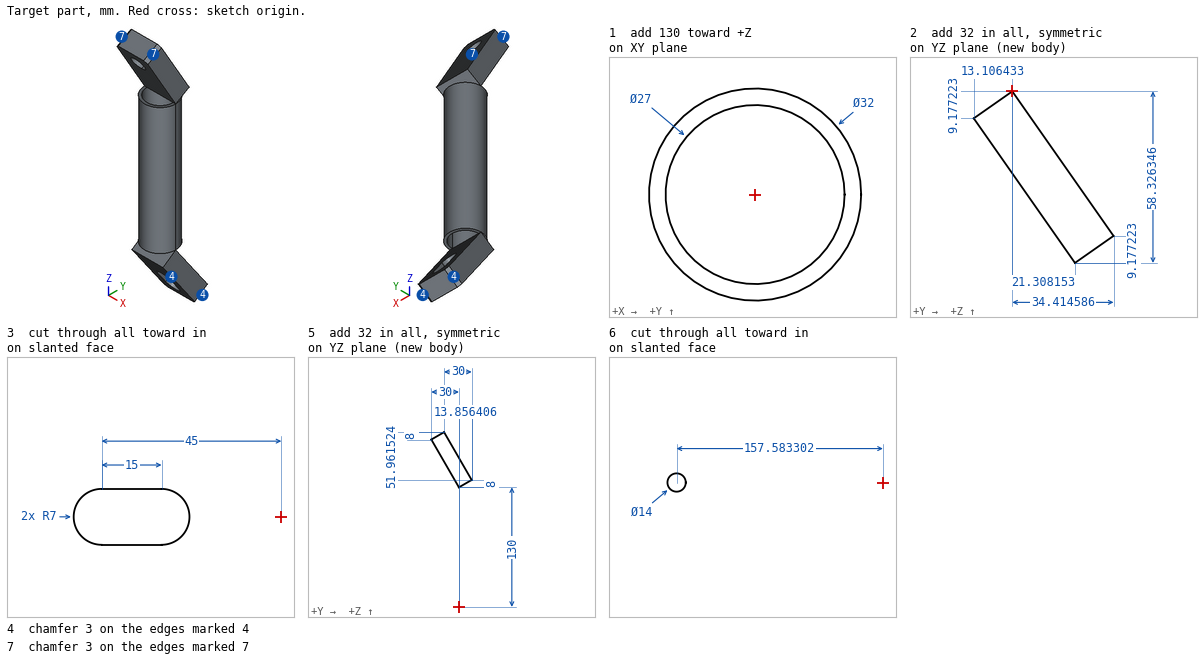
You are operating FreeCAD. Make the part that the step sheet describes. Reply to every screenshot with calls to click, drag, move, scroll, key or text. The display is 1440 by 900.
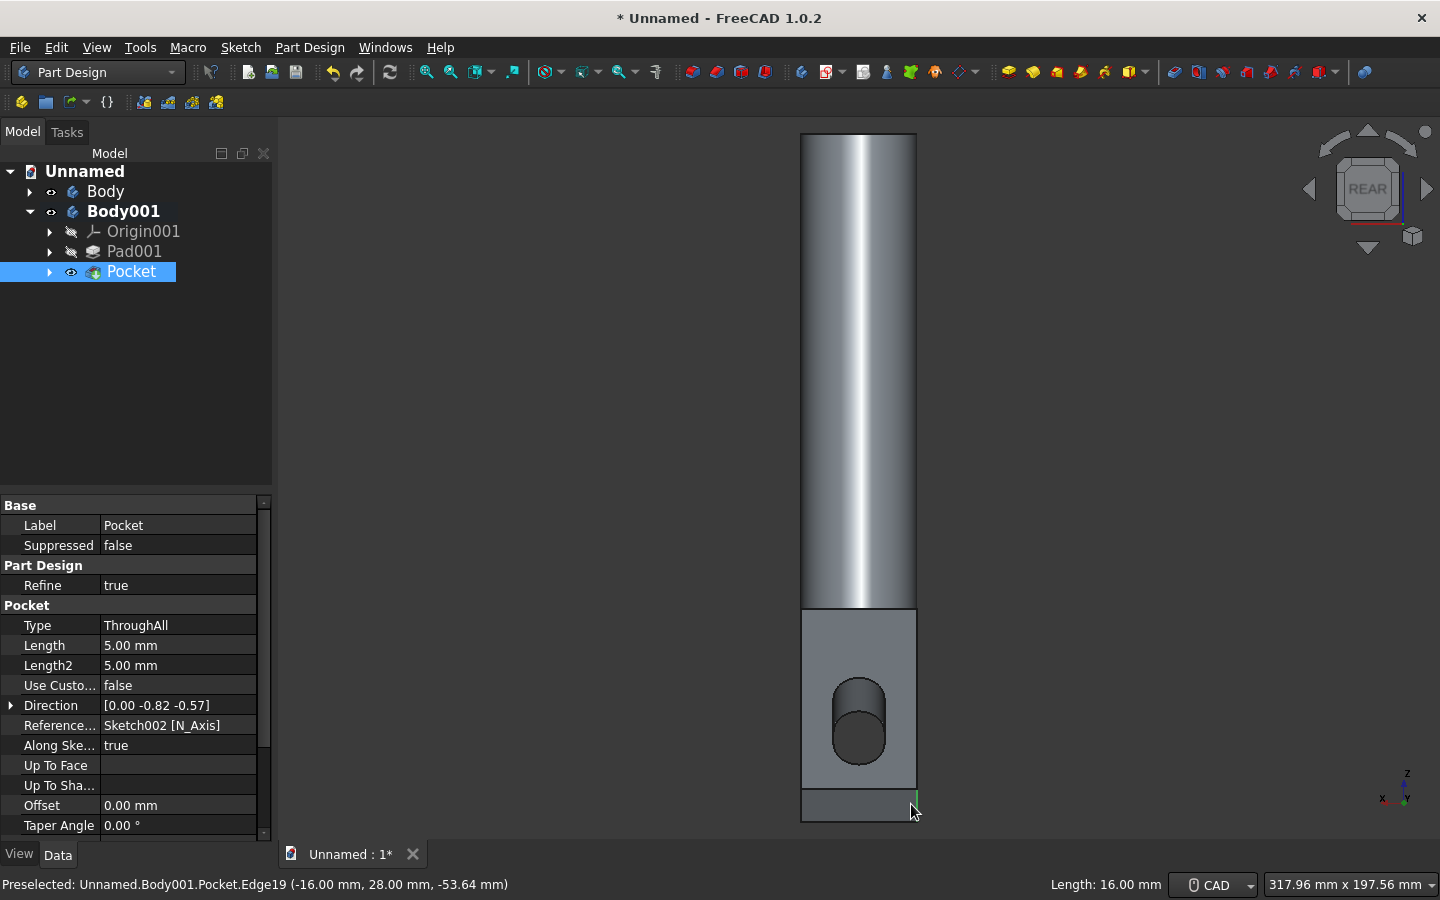
key(0)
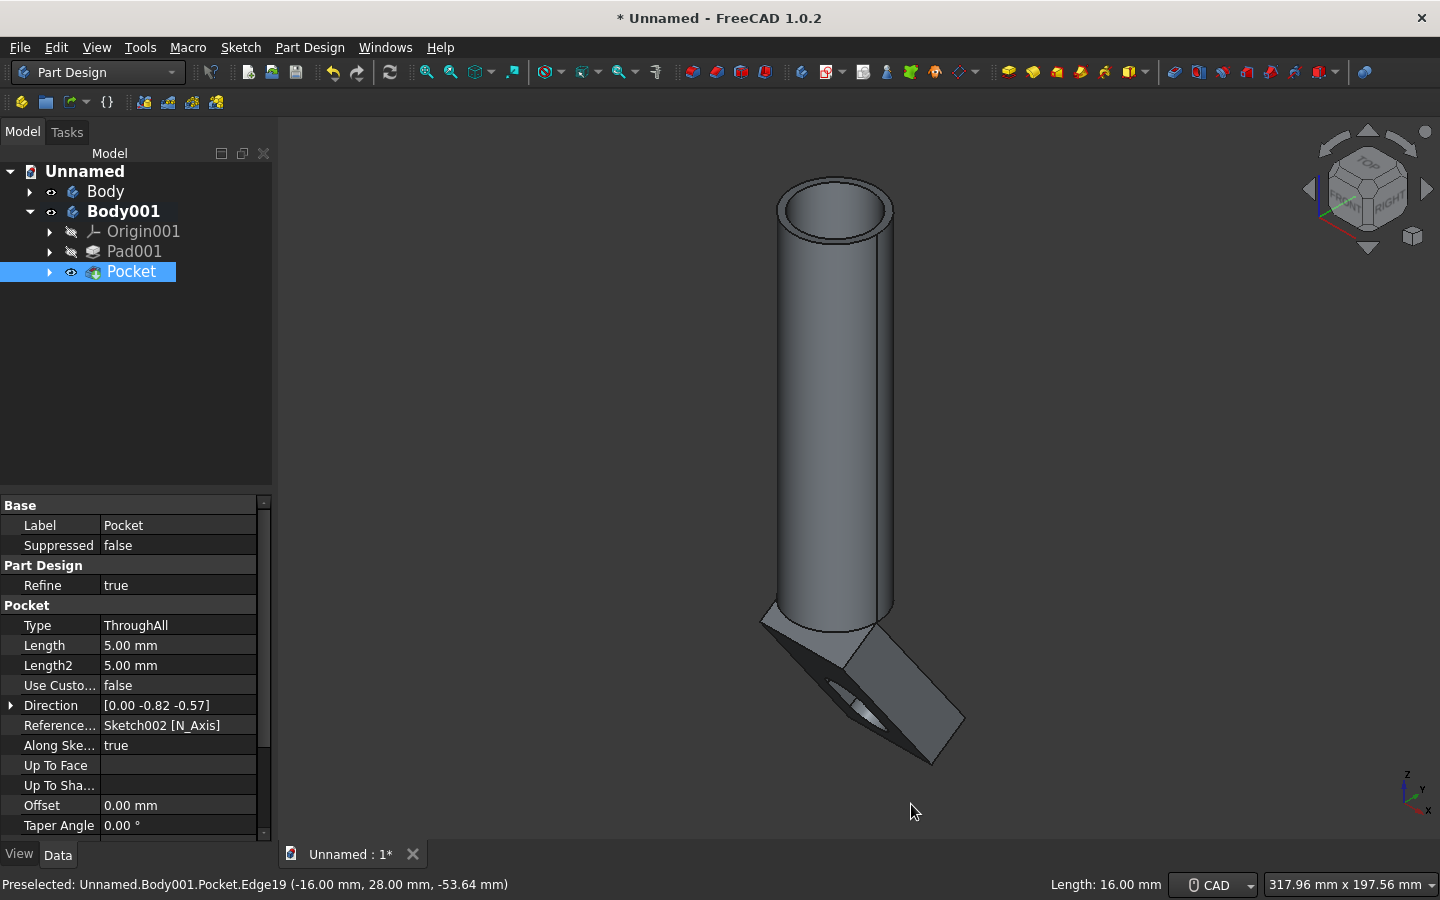
key(v)
key(f)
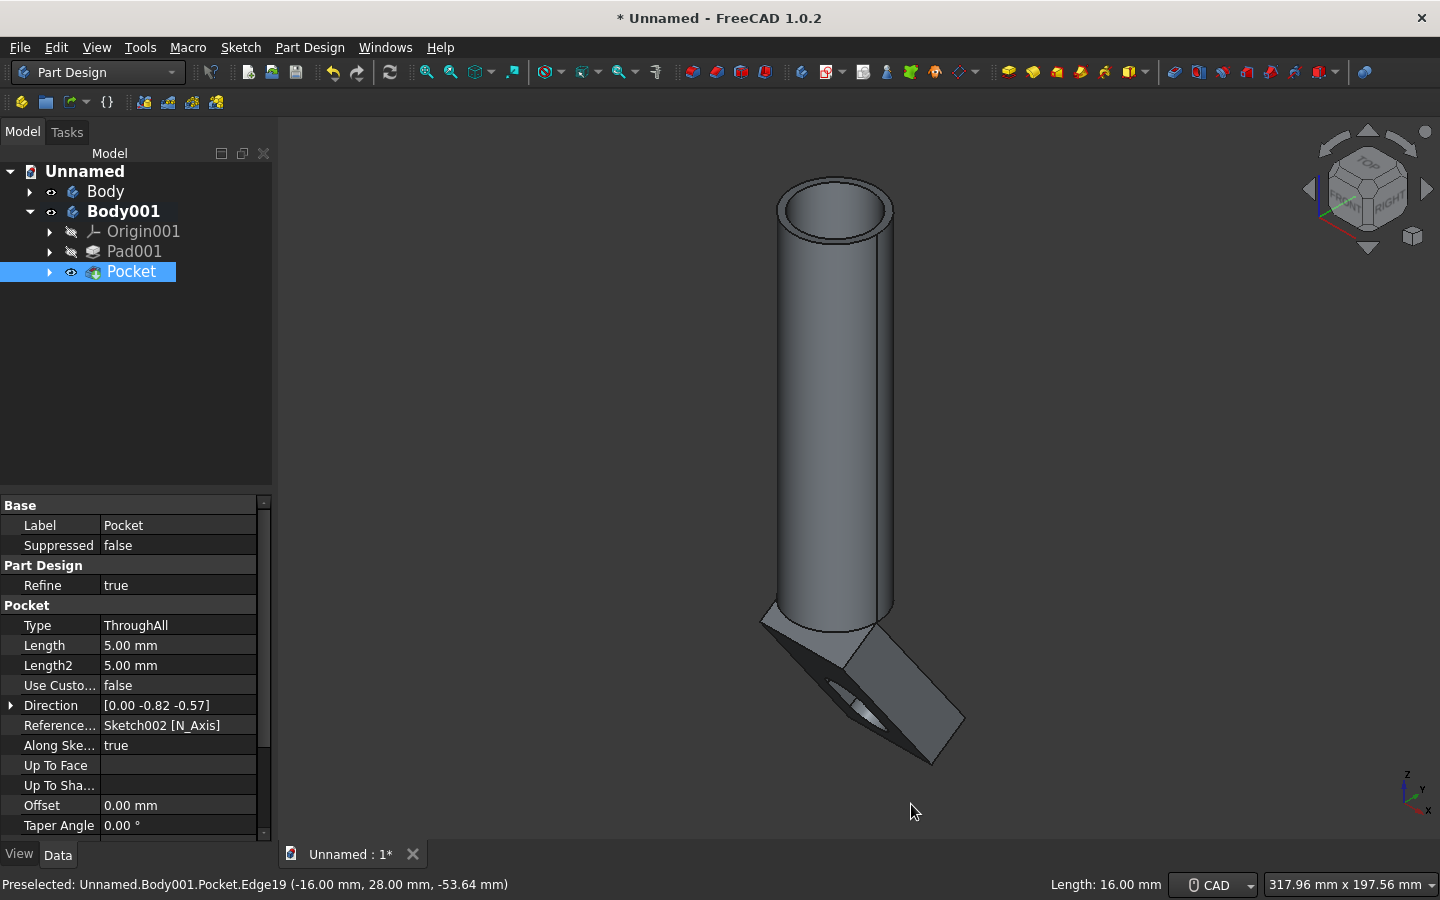
key(2)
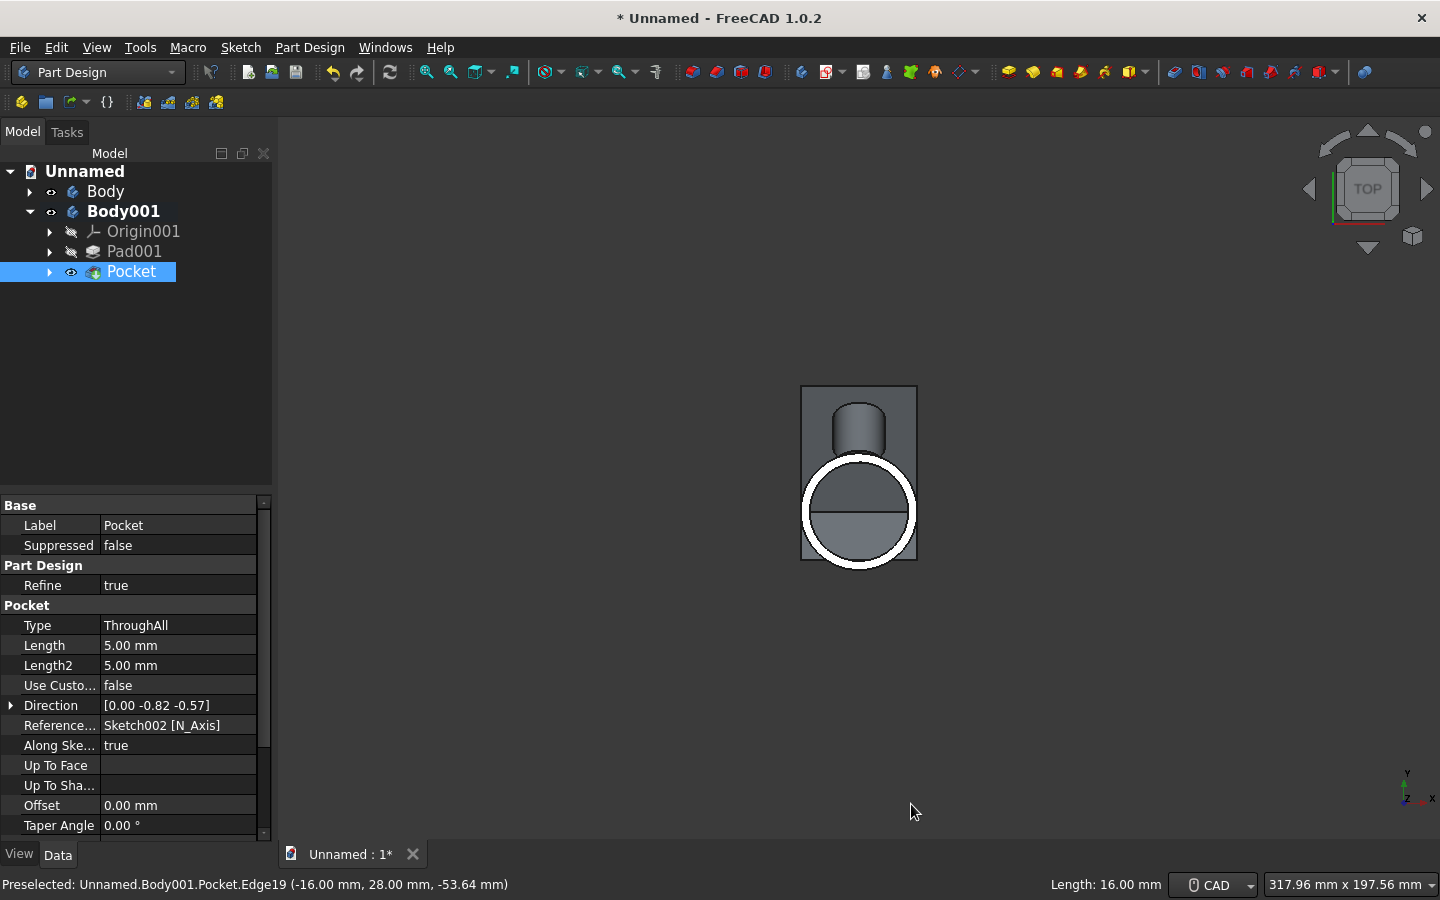
click(428, 72)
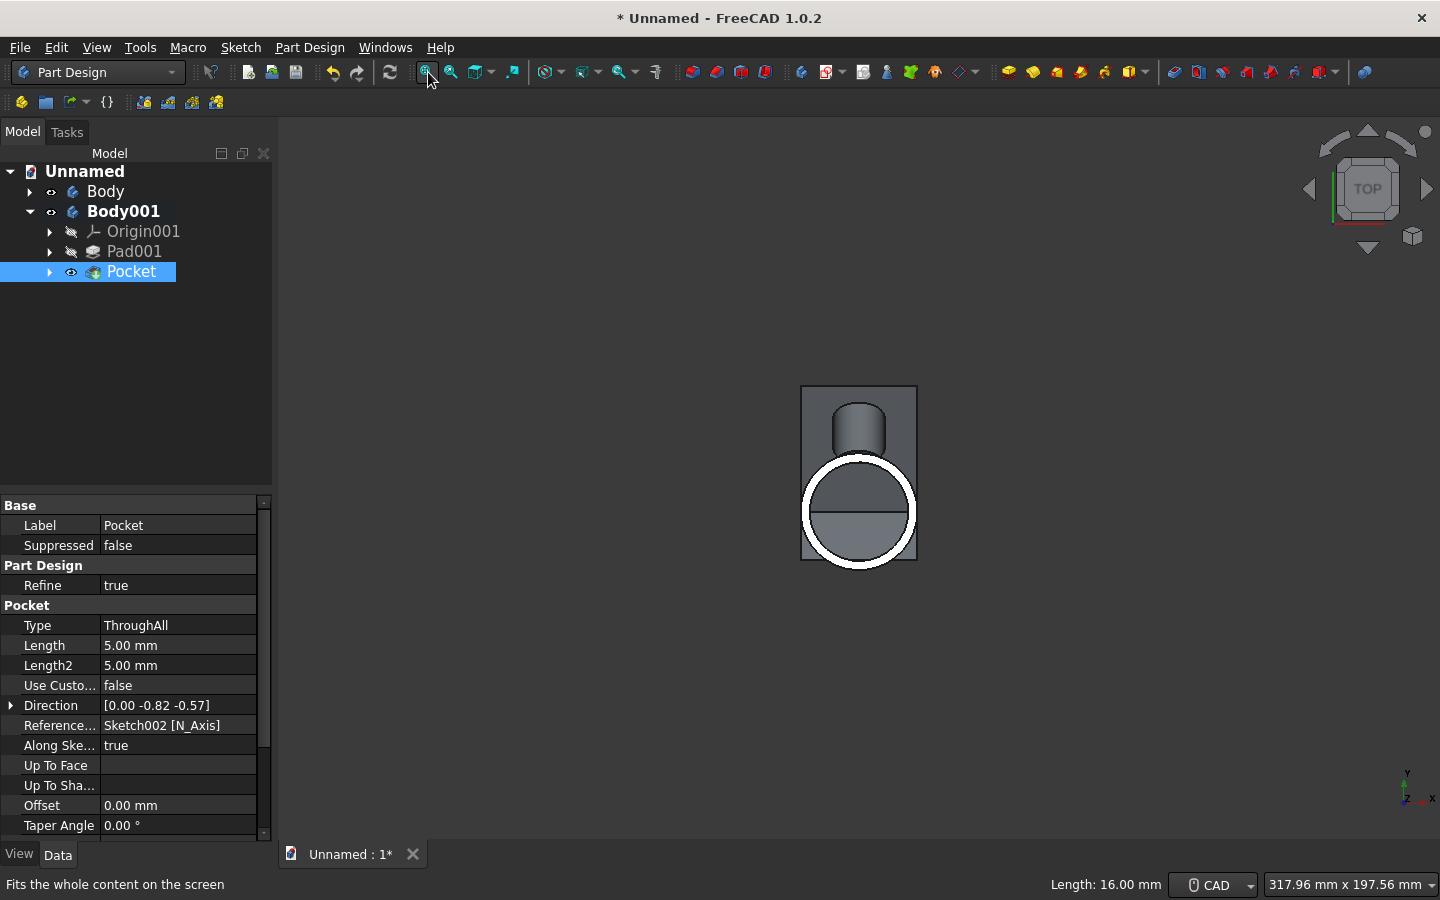
key(1)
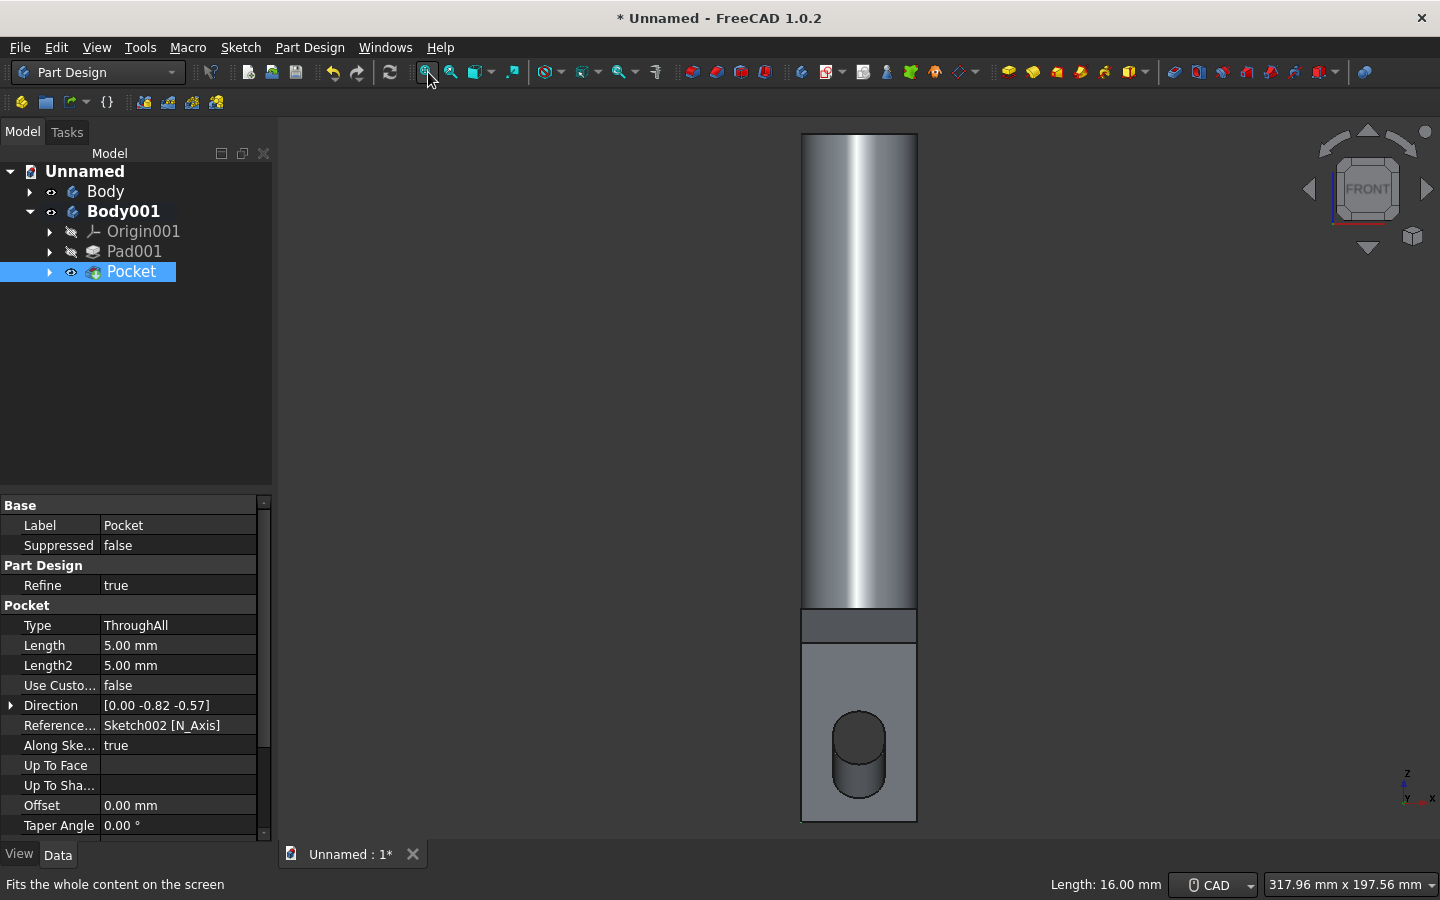
click(428, 72)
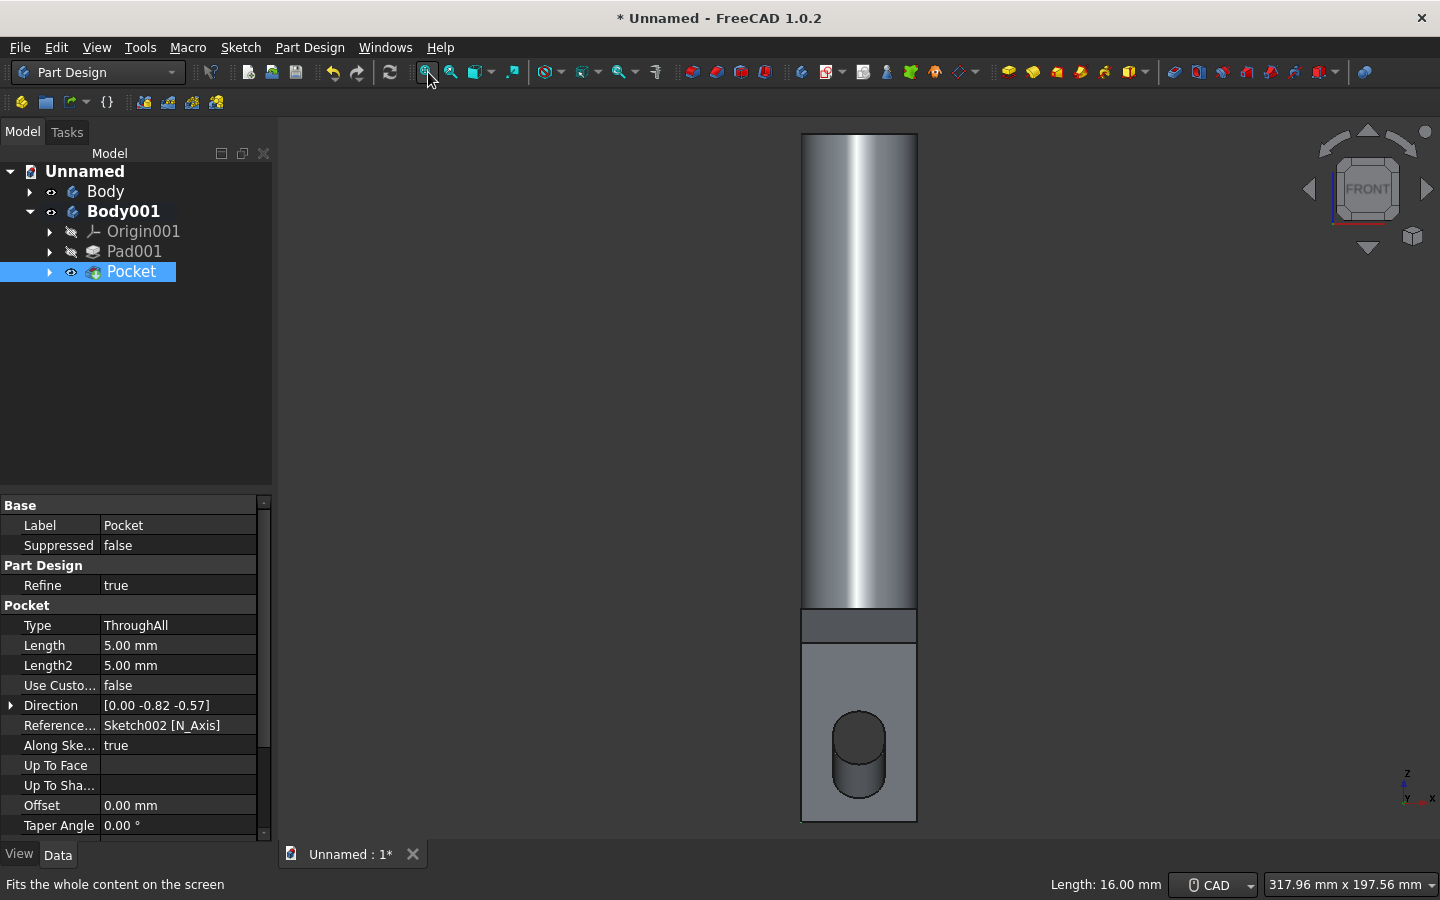
key(3)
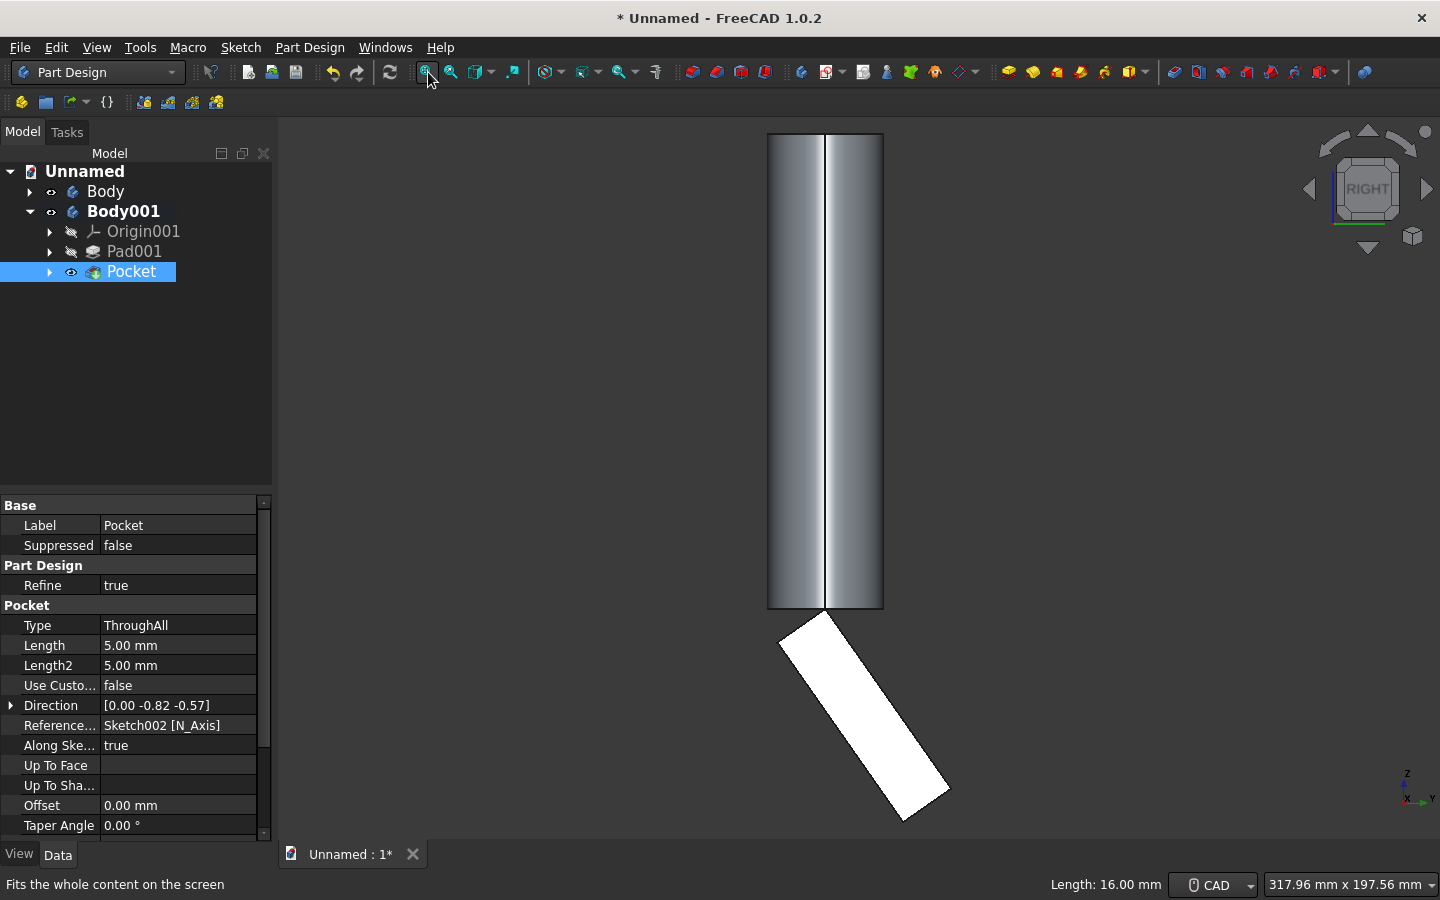
key(v)
key(f)